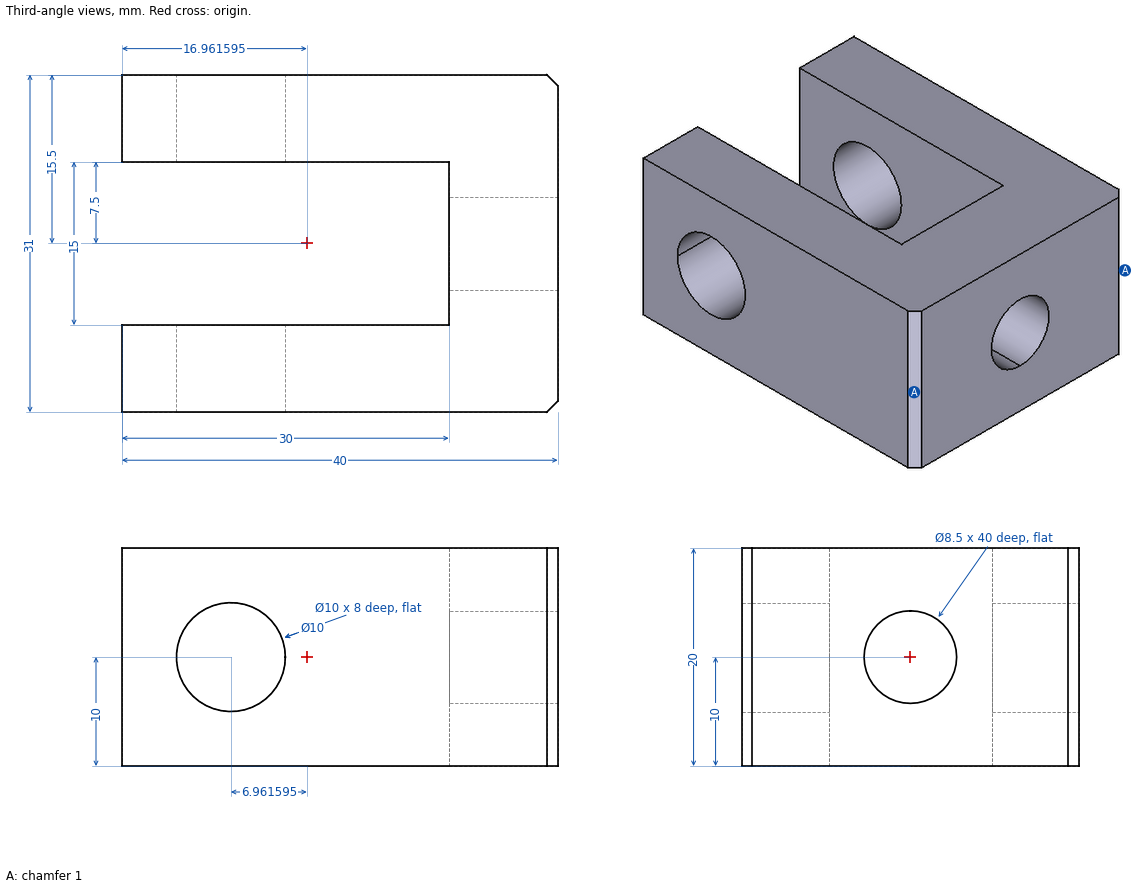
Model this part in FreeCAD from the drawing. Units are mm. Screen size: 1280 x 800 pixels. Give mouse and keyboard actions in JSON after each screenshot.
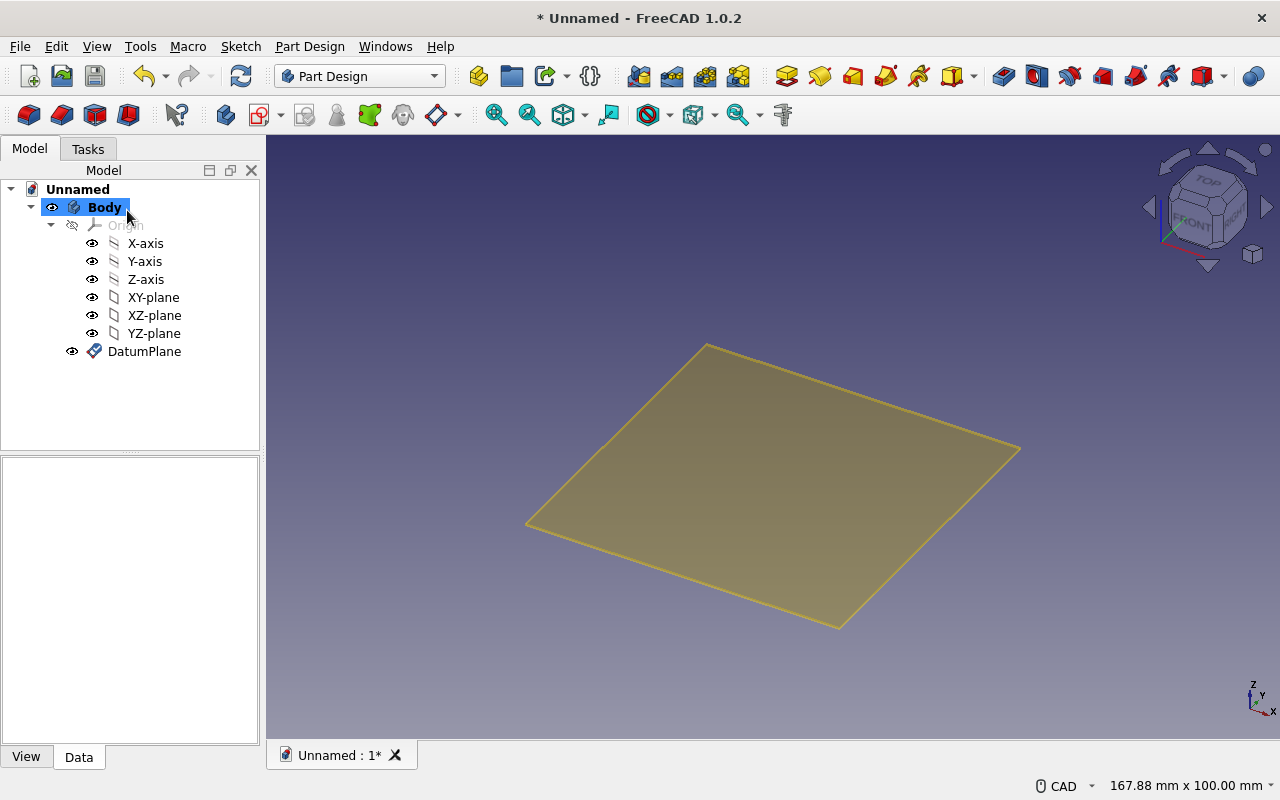
{"action": "left_click", "coordinate": [117, 351]}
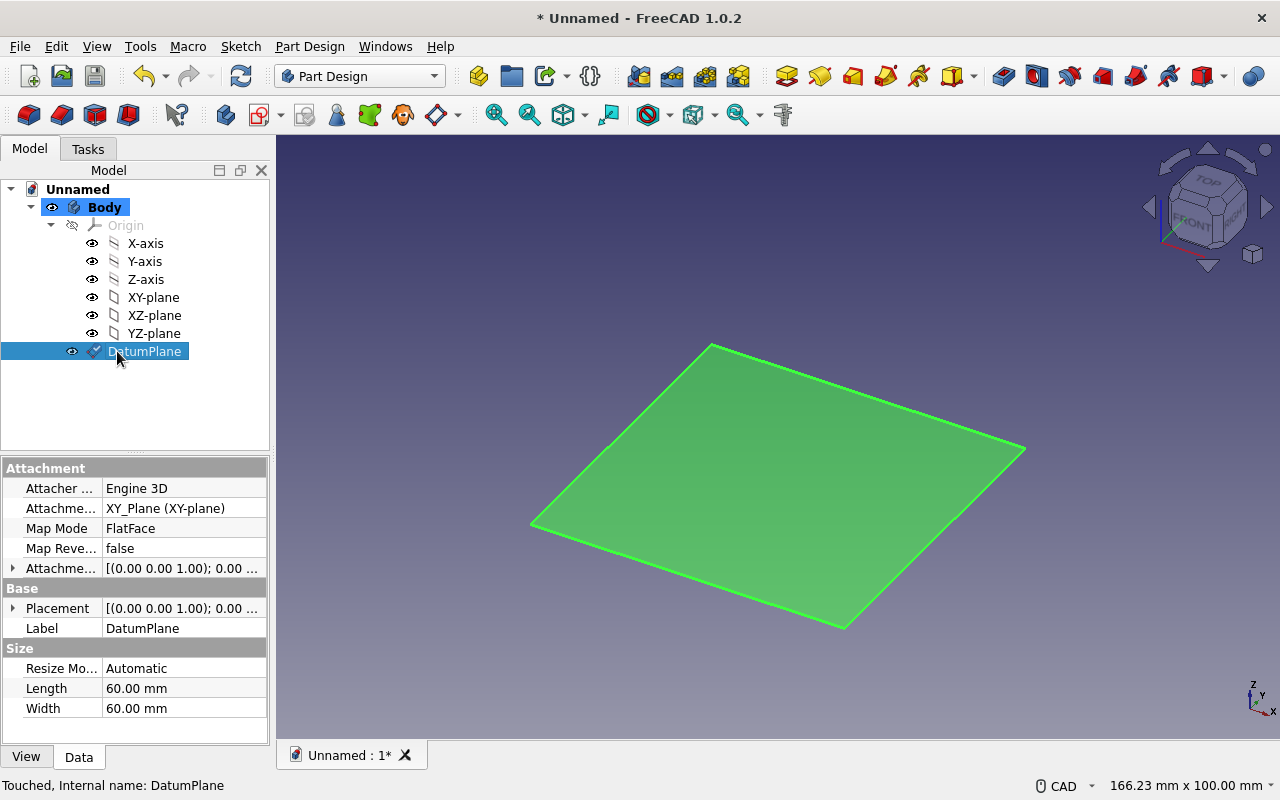
{"action": "left_click", "coordinate": [258, 116]}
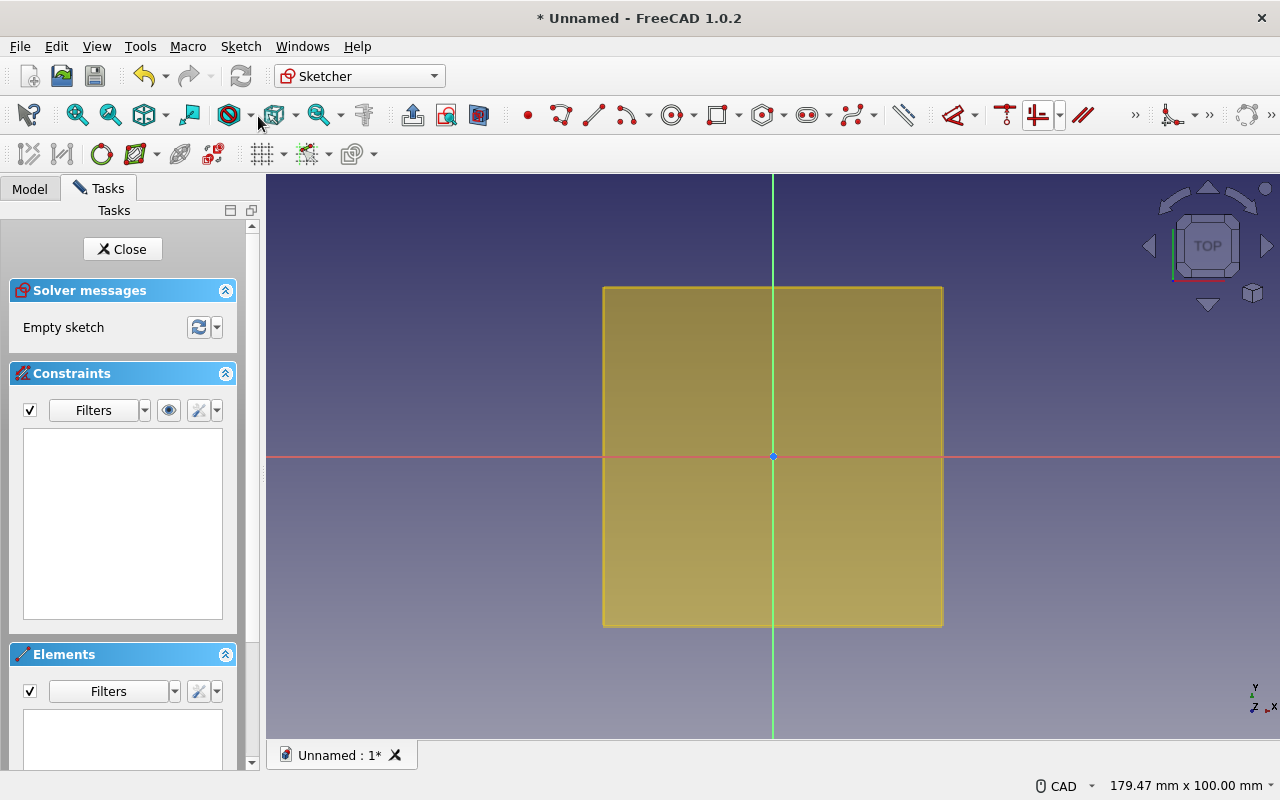
{"action": "scroll", "coordinate": [860, 456], "scroll_direction": "up", "scroll_amount": 4}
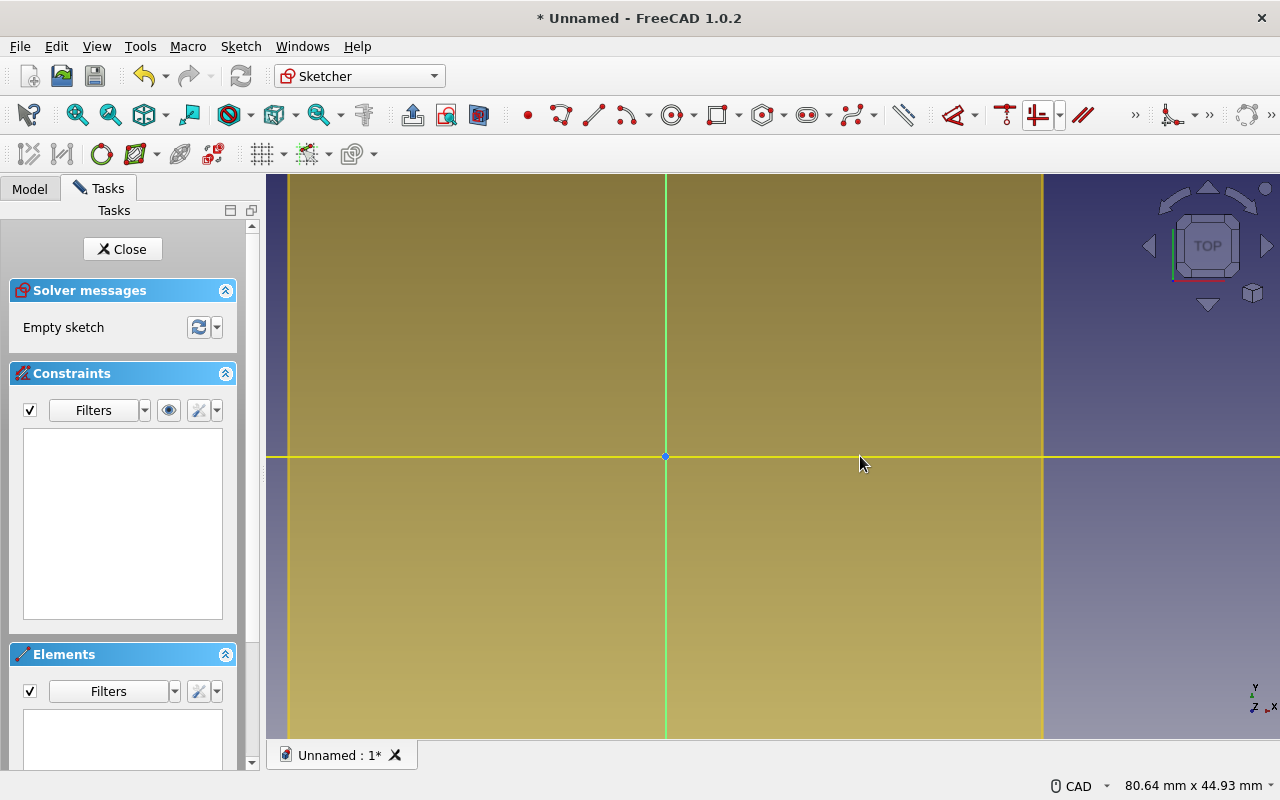
{"action": "left_click", "coordinate": [716, 116]}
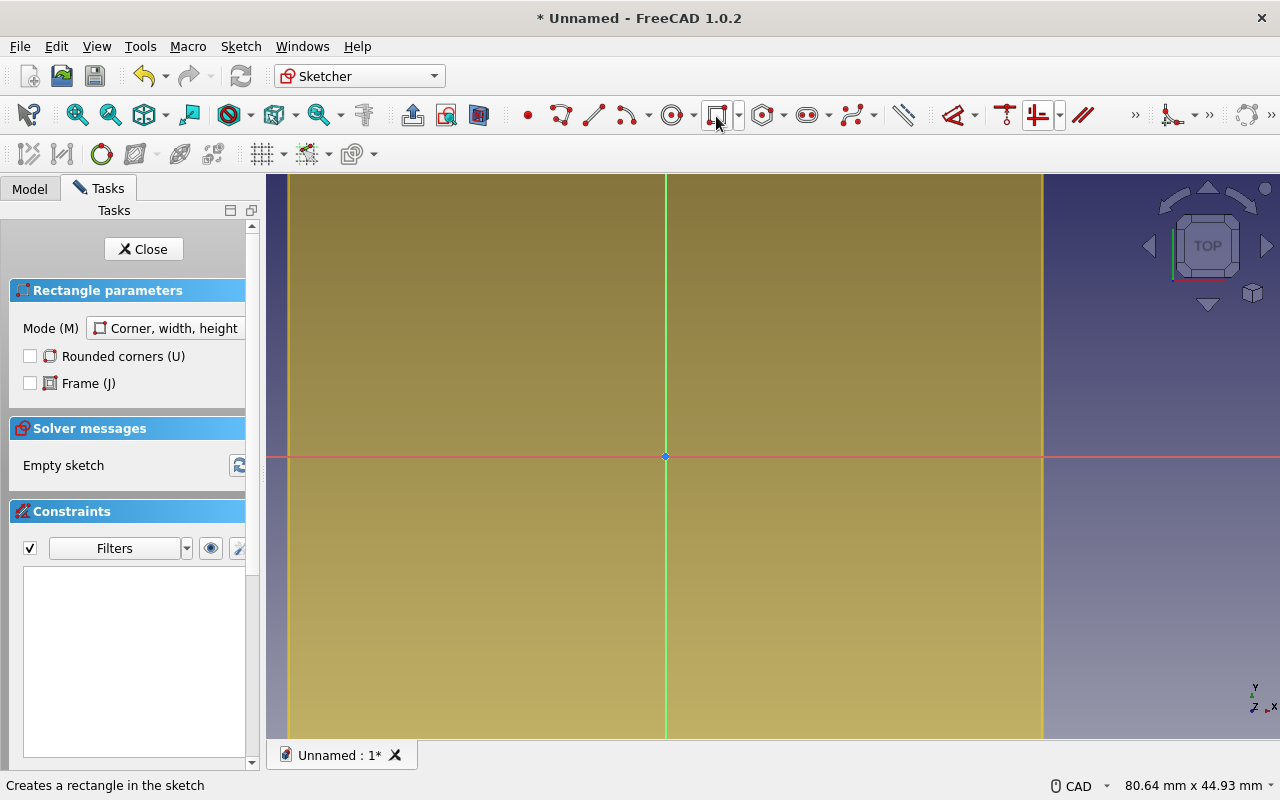
{"action": "left_click", "coordinate": [452, 262]}
{"action": "left_click", "coordinate": [955, 651]}
{"action": "key", "text": "Escape"}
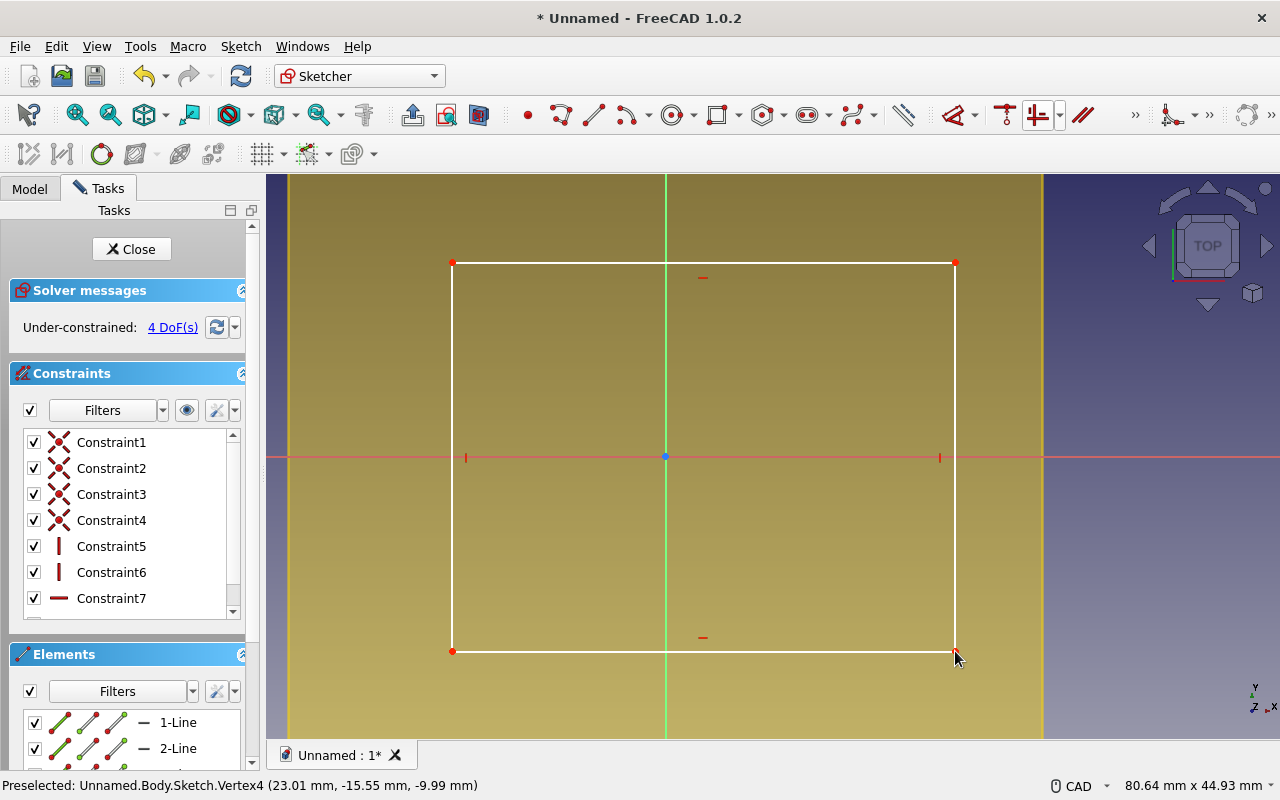
{"action": "key", "text": "d"}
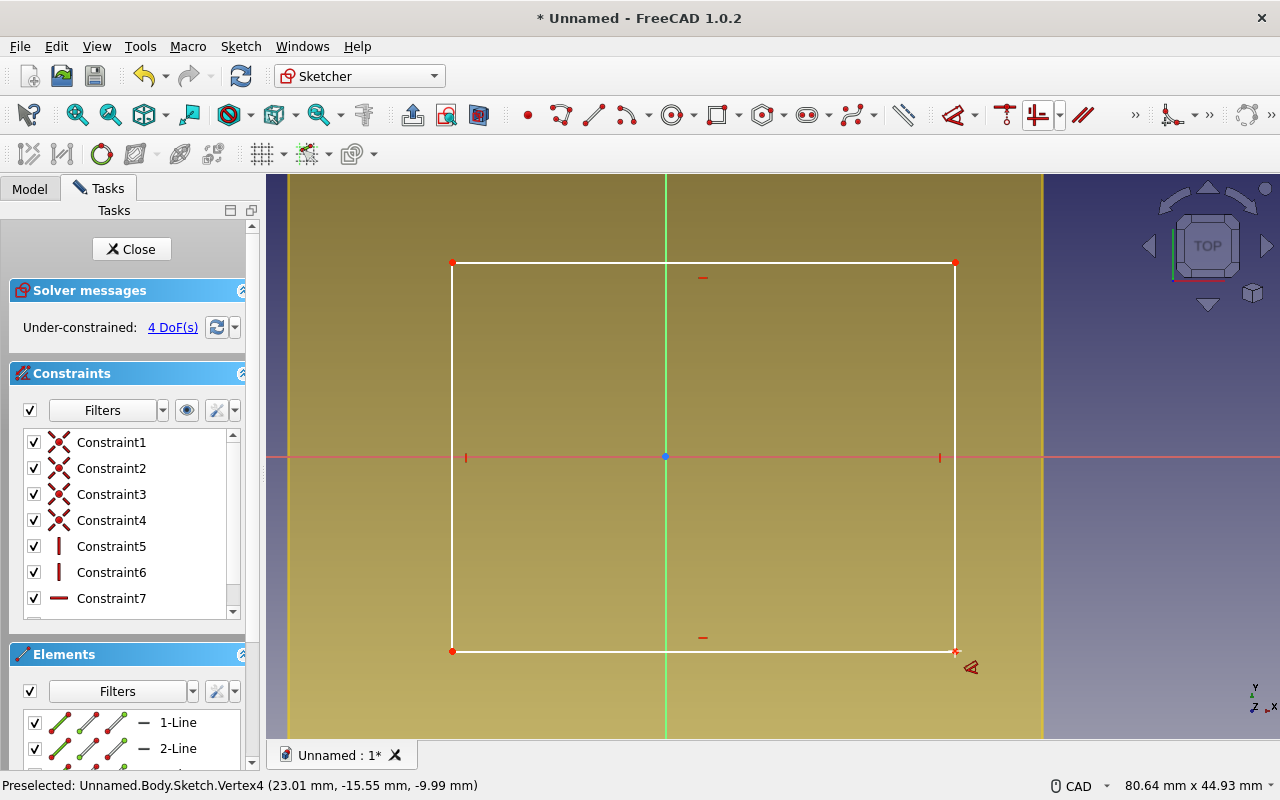
{"action": "left_click", "coordinate": [452, 380]}
{"action": "left_click", "coordinate": [418, 368]}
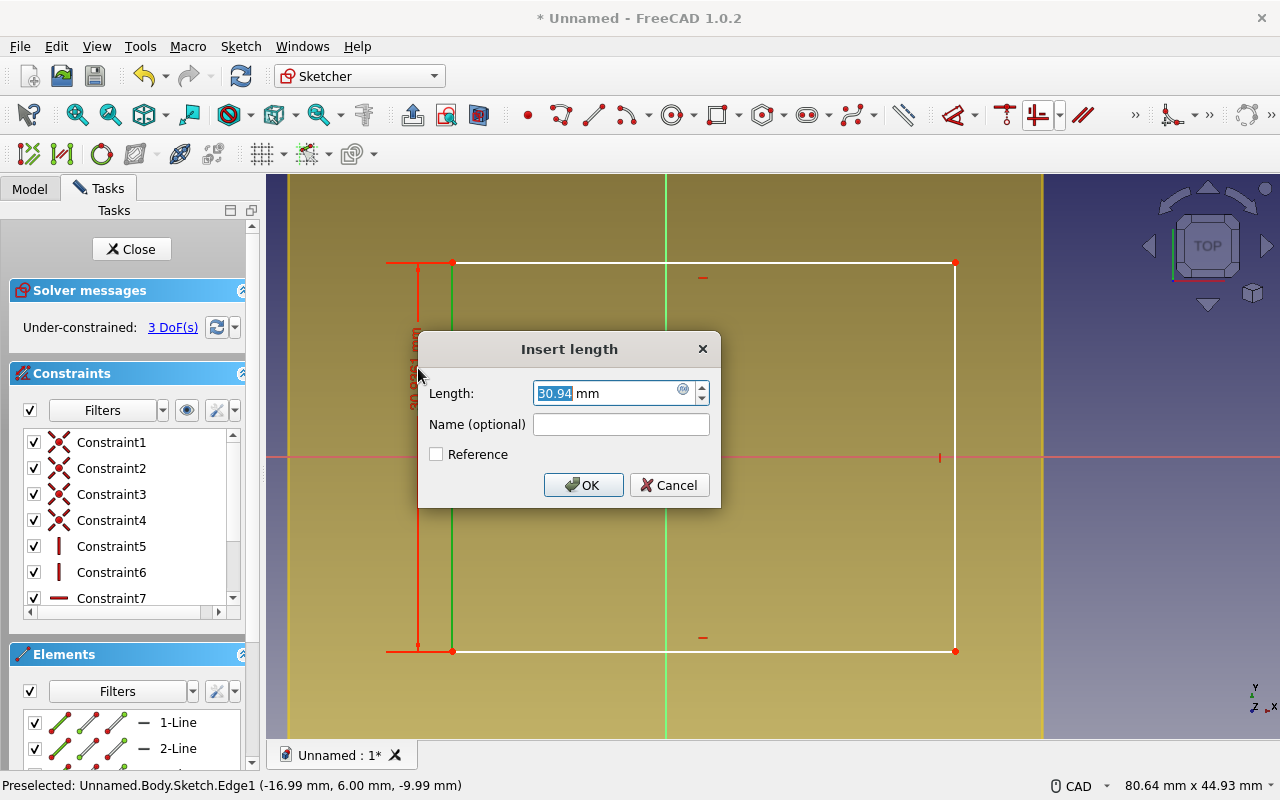
{"action": "type", "text": "31"}
{"action": "key", "text": "Return"}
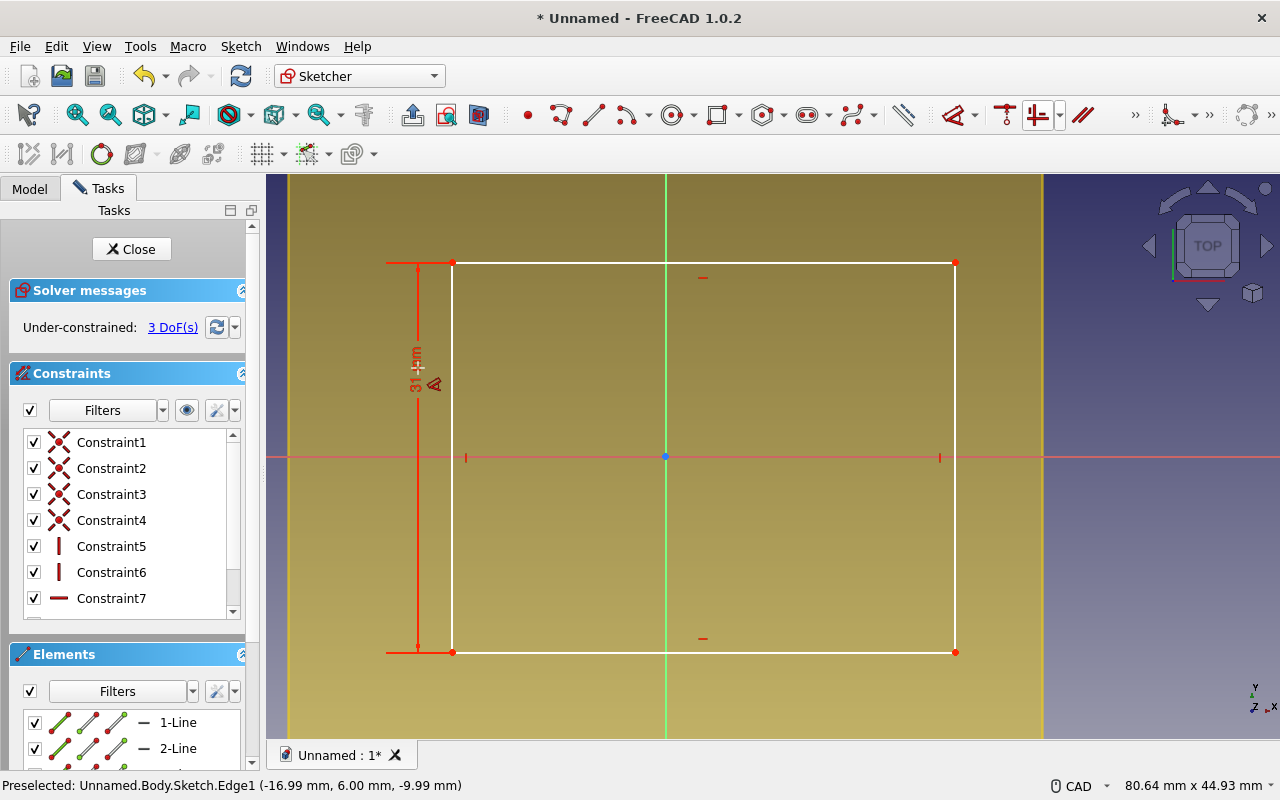
{"action": "left_click", "coordinate": [603, 653]}
{"action": "left_click", "coordinate": [704, 687]}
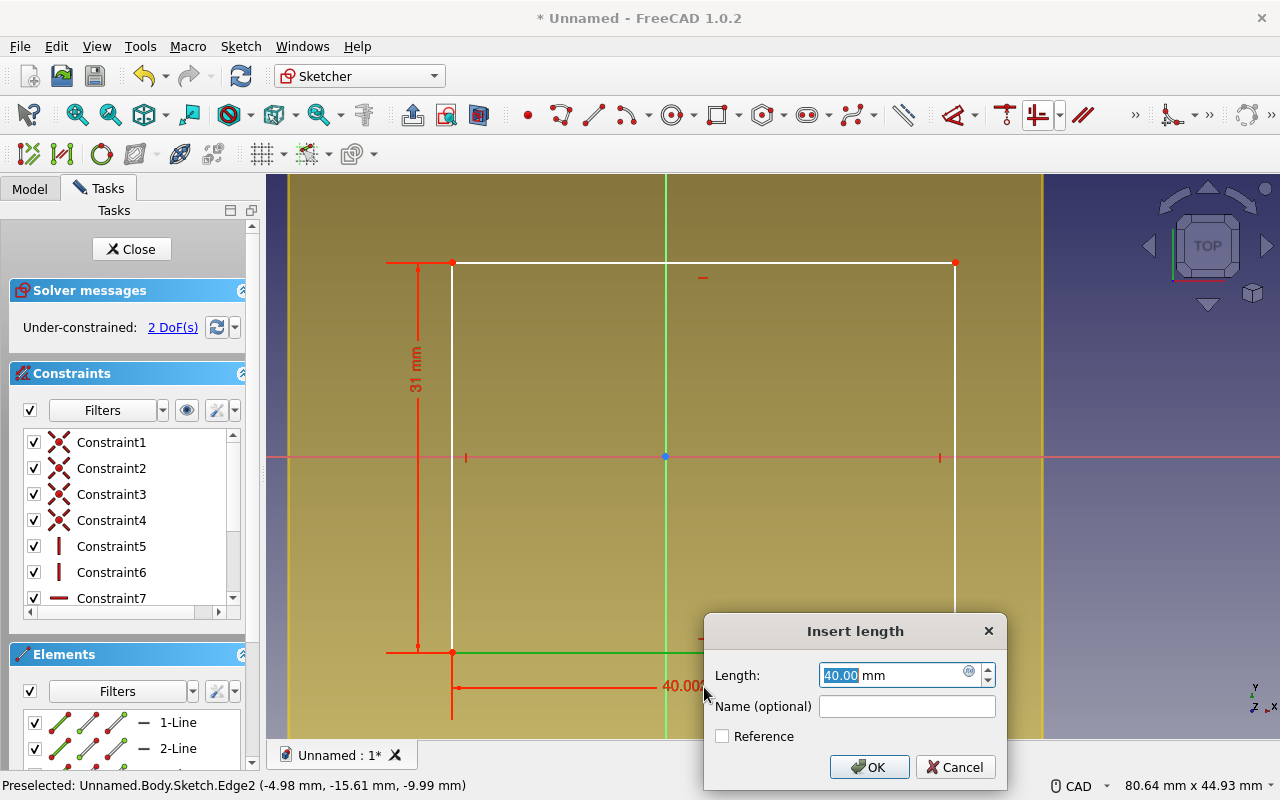
{"action": "type", "text": "40"}
{"action": "key", "text": "Return"}